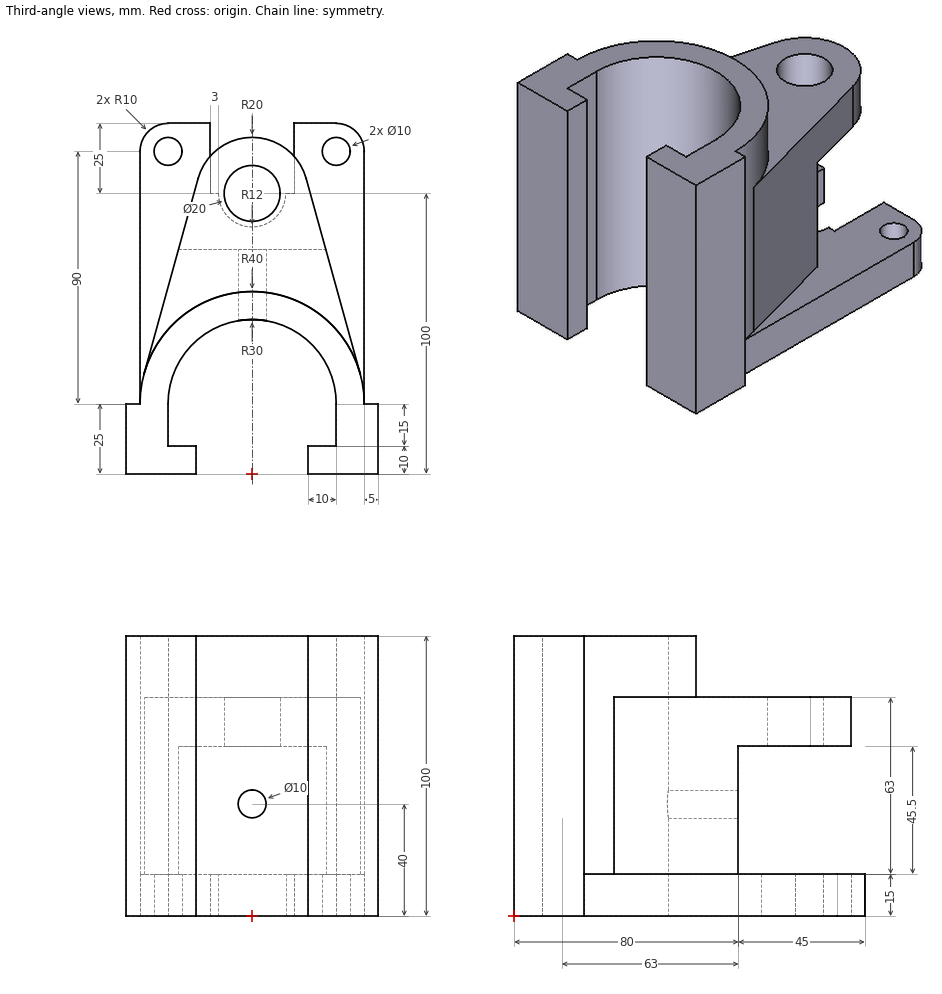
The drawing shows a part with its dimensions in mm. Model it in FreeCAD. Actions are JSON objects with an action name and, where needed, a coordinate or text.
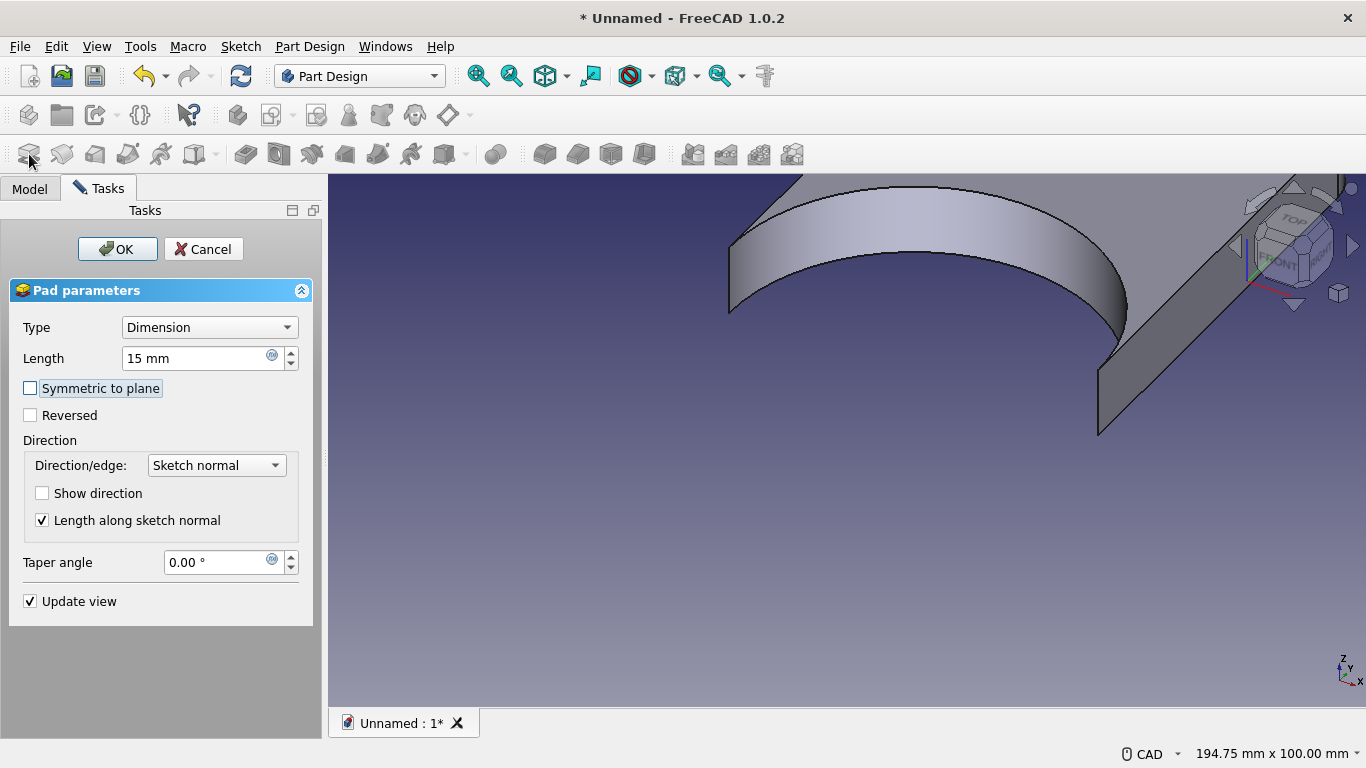
{"action": "left_click", "coordinate": [118, 249]}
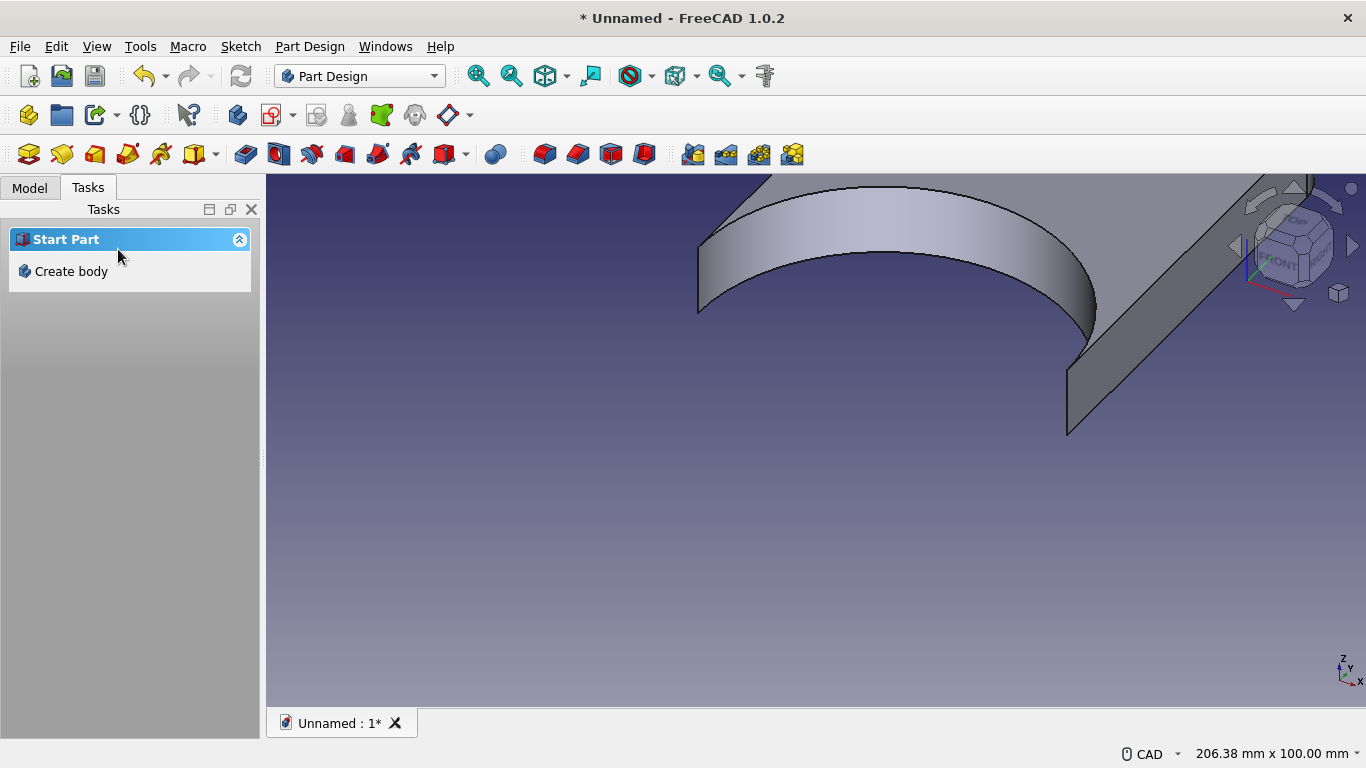
{"action": "key", "text": "v f"}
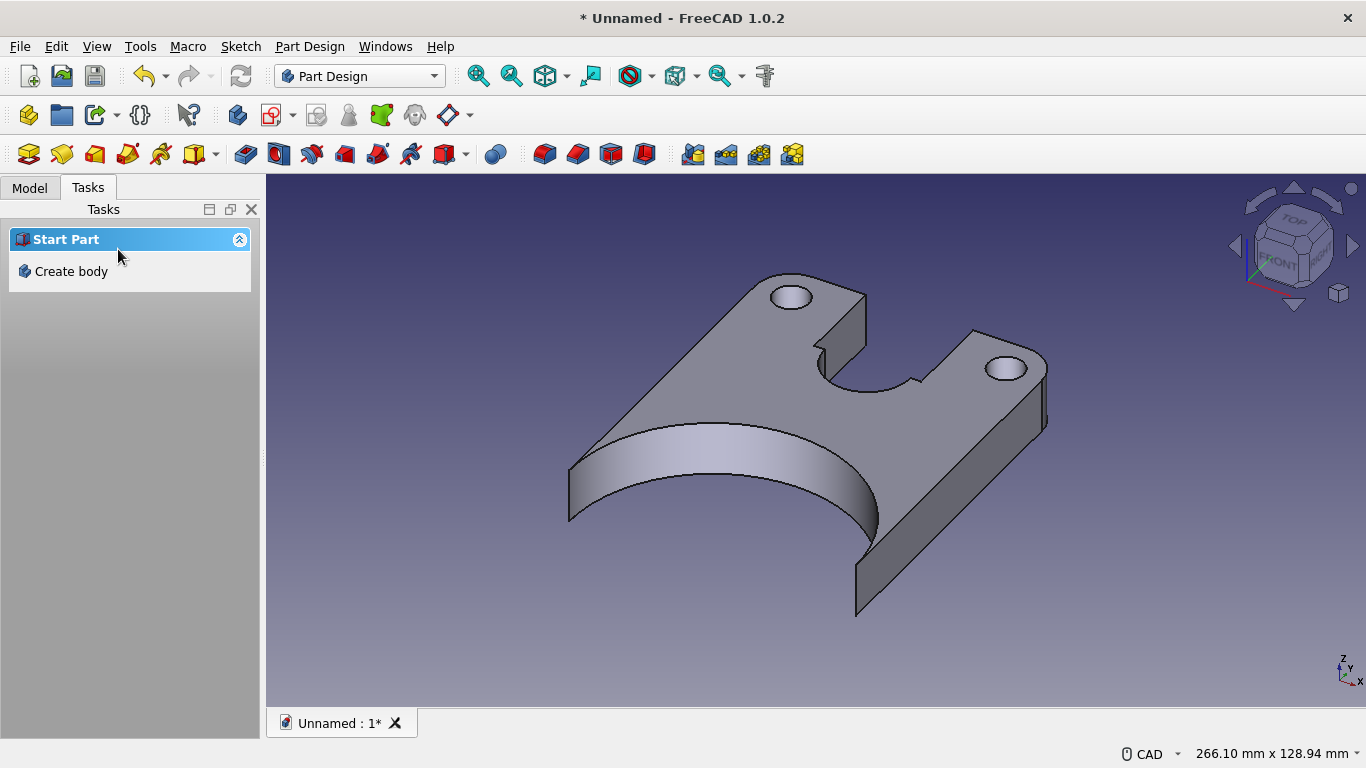
{"action": "key", "text": "5"}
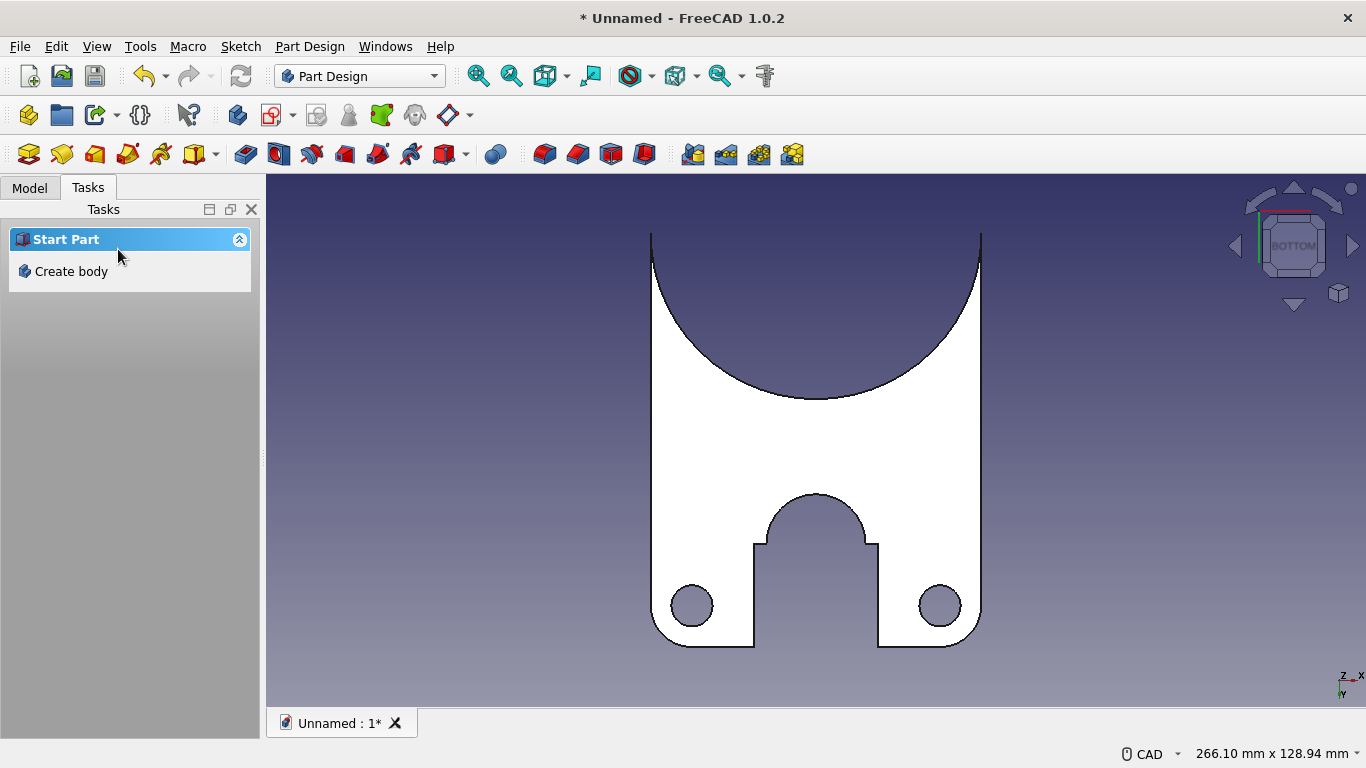
{"action": "left_click", "coordinate": [910, 439]}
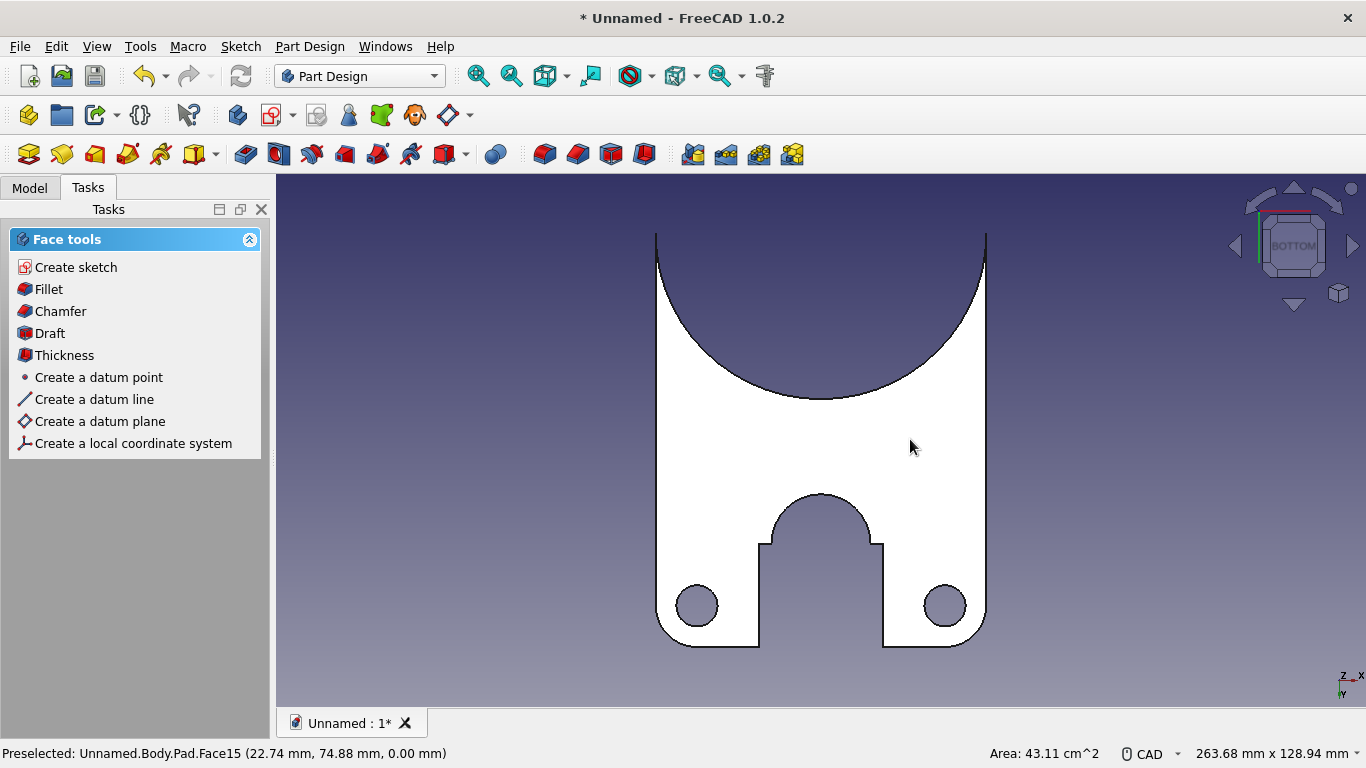
{"action": "left_click", "coordinate": [270, 116]}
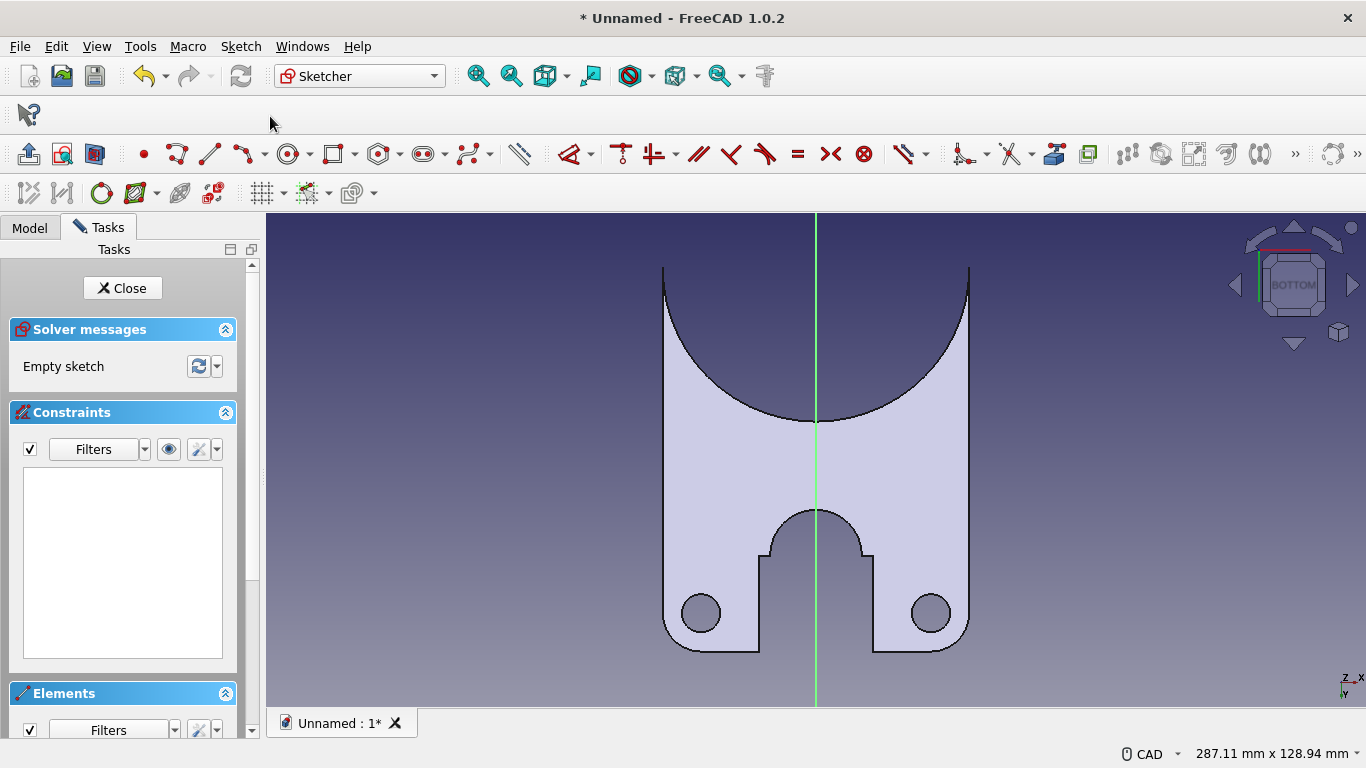
{"action": "scroll", "coordinate": [608, 679], "scroll_direction": "down", "scroll_amount": 2}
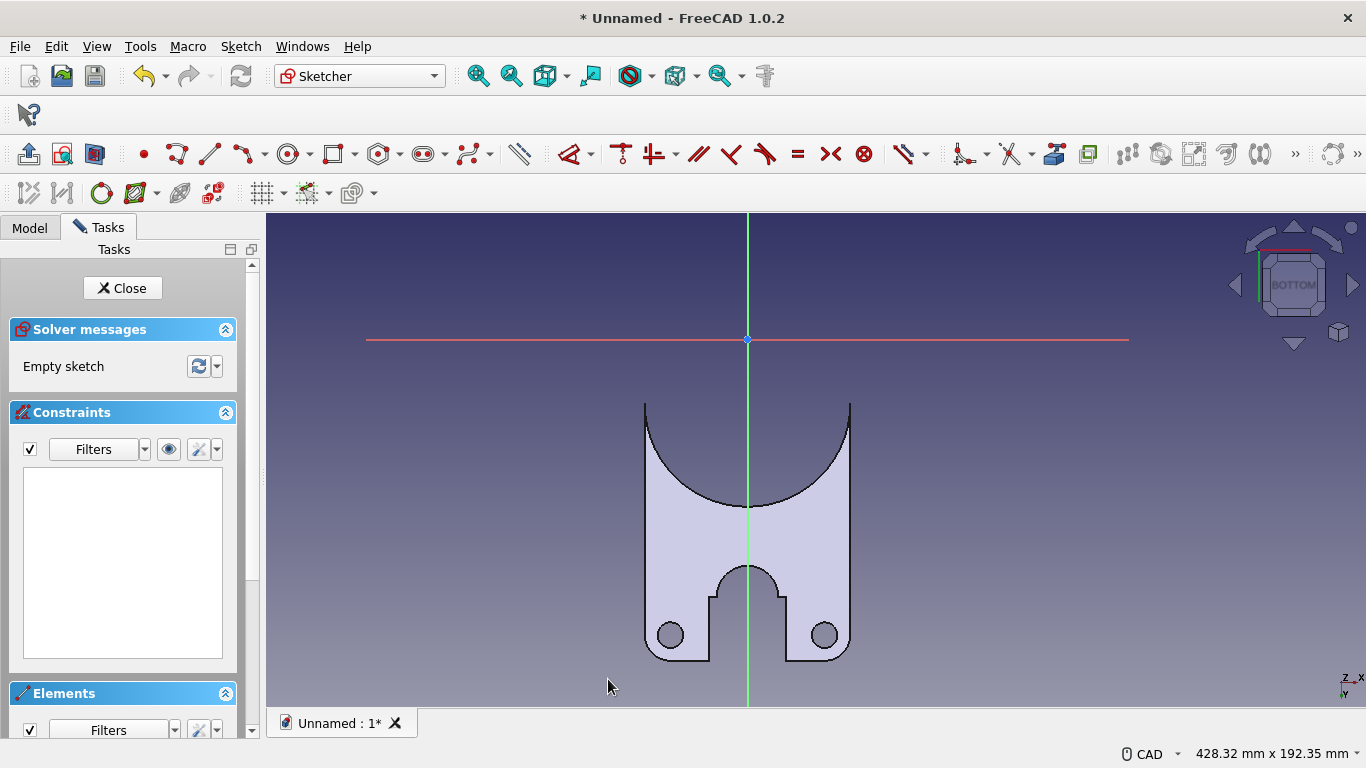
{"action": "scroll", "coordinate": [748, 379], "scroll_direction": "up", "scroll_amount": 3}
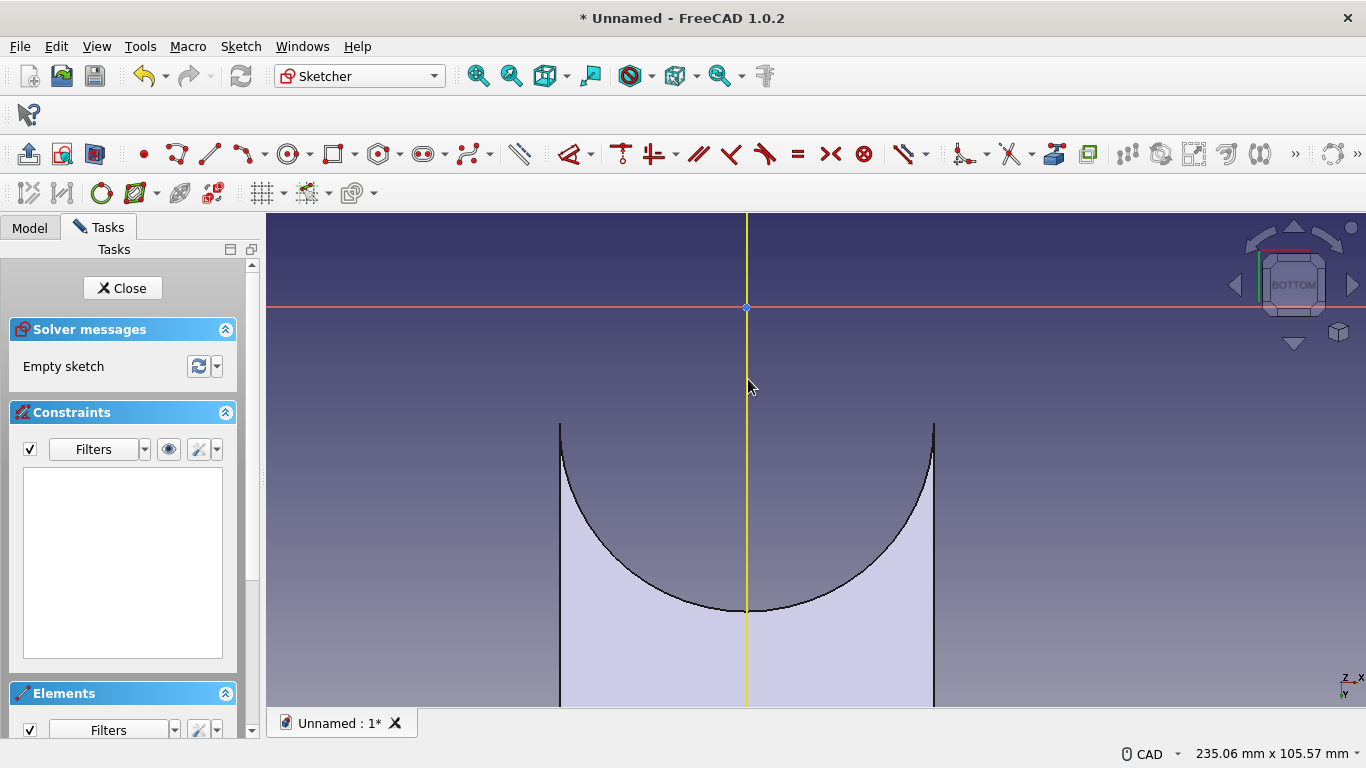
{"action": "left_click", "coordinate": [177, 154]}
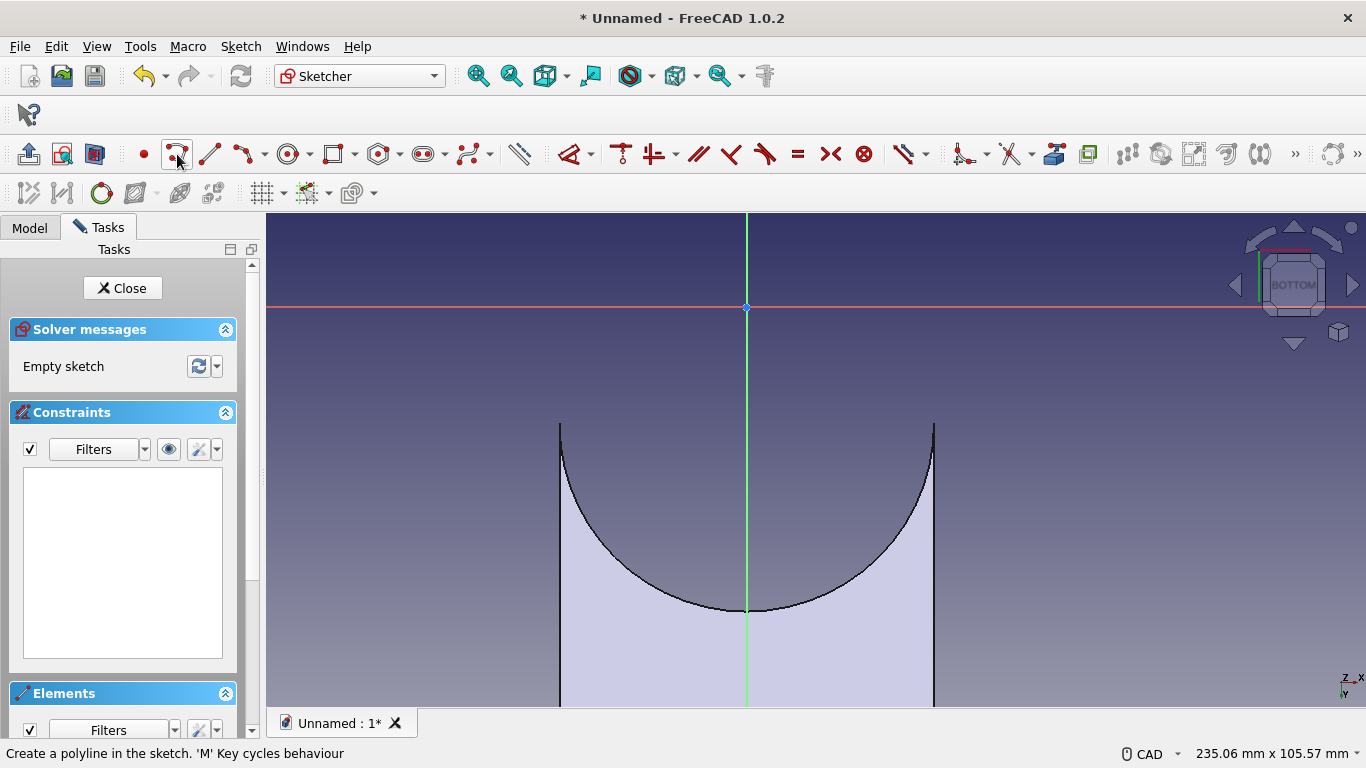
{"action": "left_click", "coordinate": [887, 424]}
{"action": "left_click", "coordinate": [887, 354]}
{"action": "left_click", "coordinate": [840, 354]}
{"action": "left_click", "coordinate": [840, 307]}
{"action": "left_click", "coordinate": [957, 316]}
{"action": "left_click", "coordinate": [957, 424]}
{"action": "left_click", "coordinate": [934, 424]}
{"action": "right_click", "coordinate": [934, 424]}